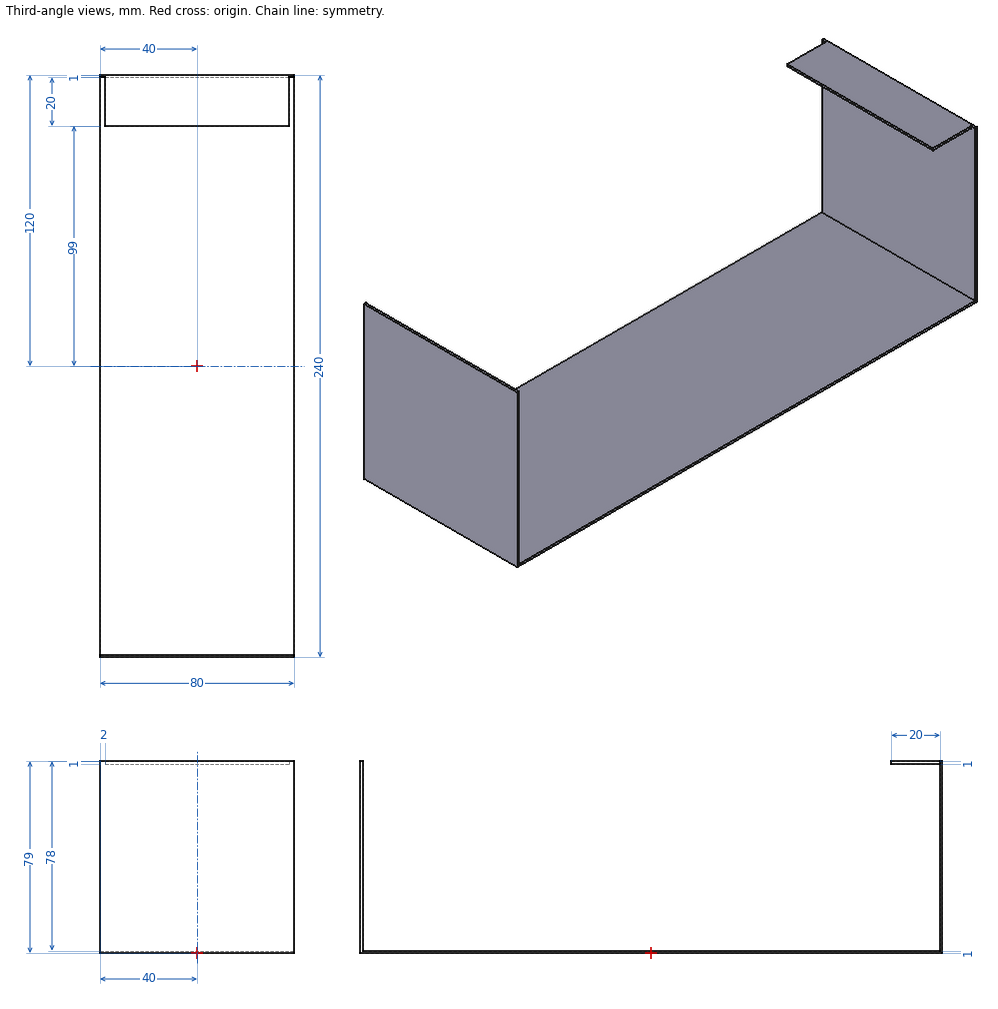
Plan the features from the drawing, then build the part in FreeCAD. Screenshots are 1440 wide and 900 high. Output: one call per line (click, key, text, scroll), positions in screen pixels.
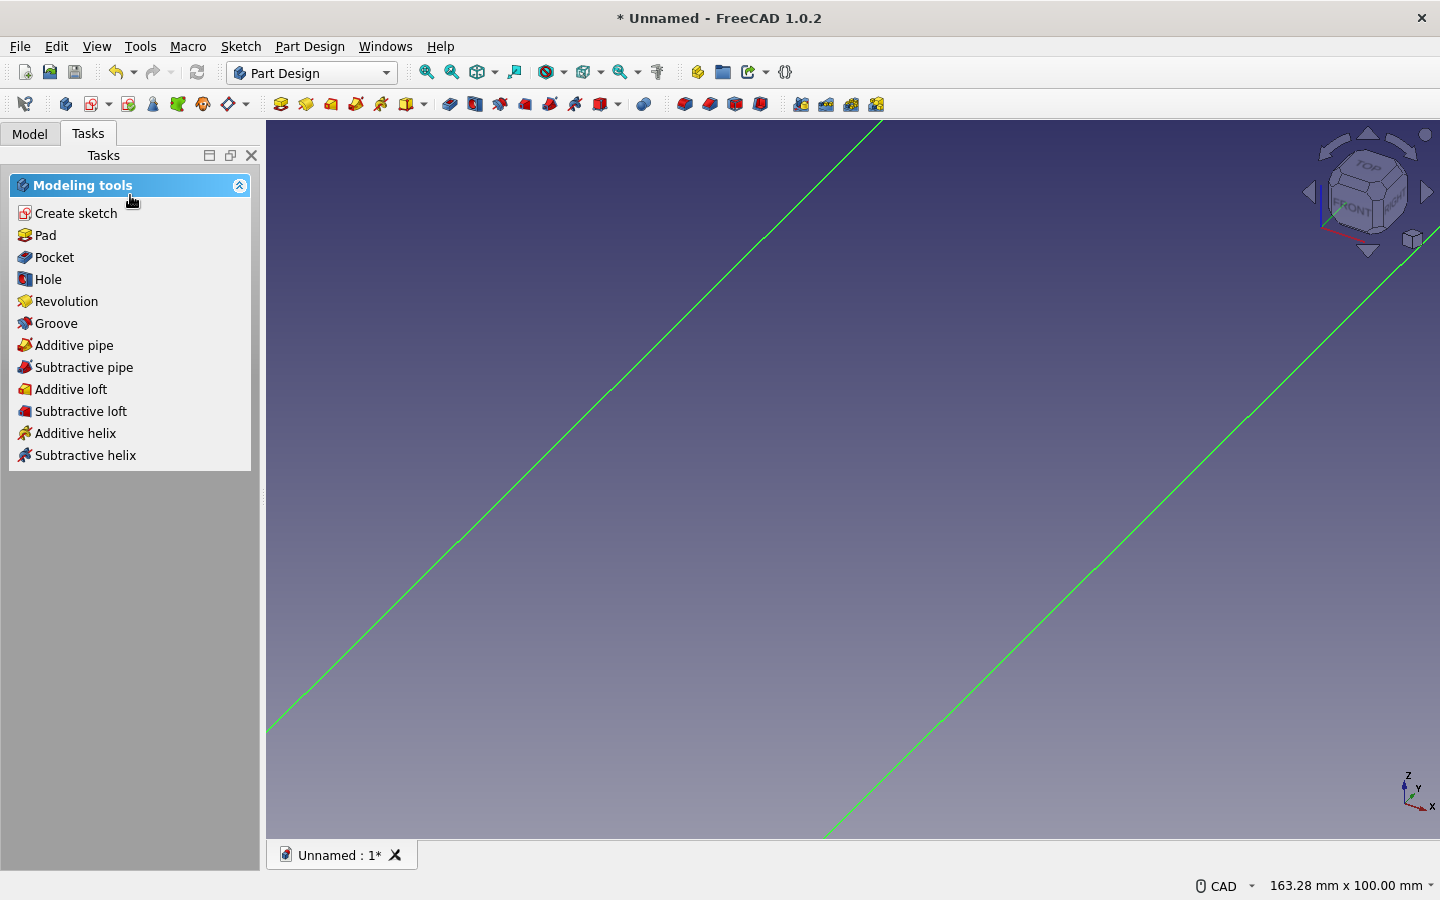
click(281, 104)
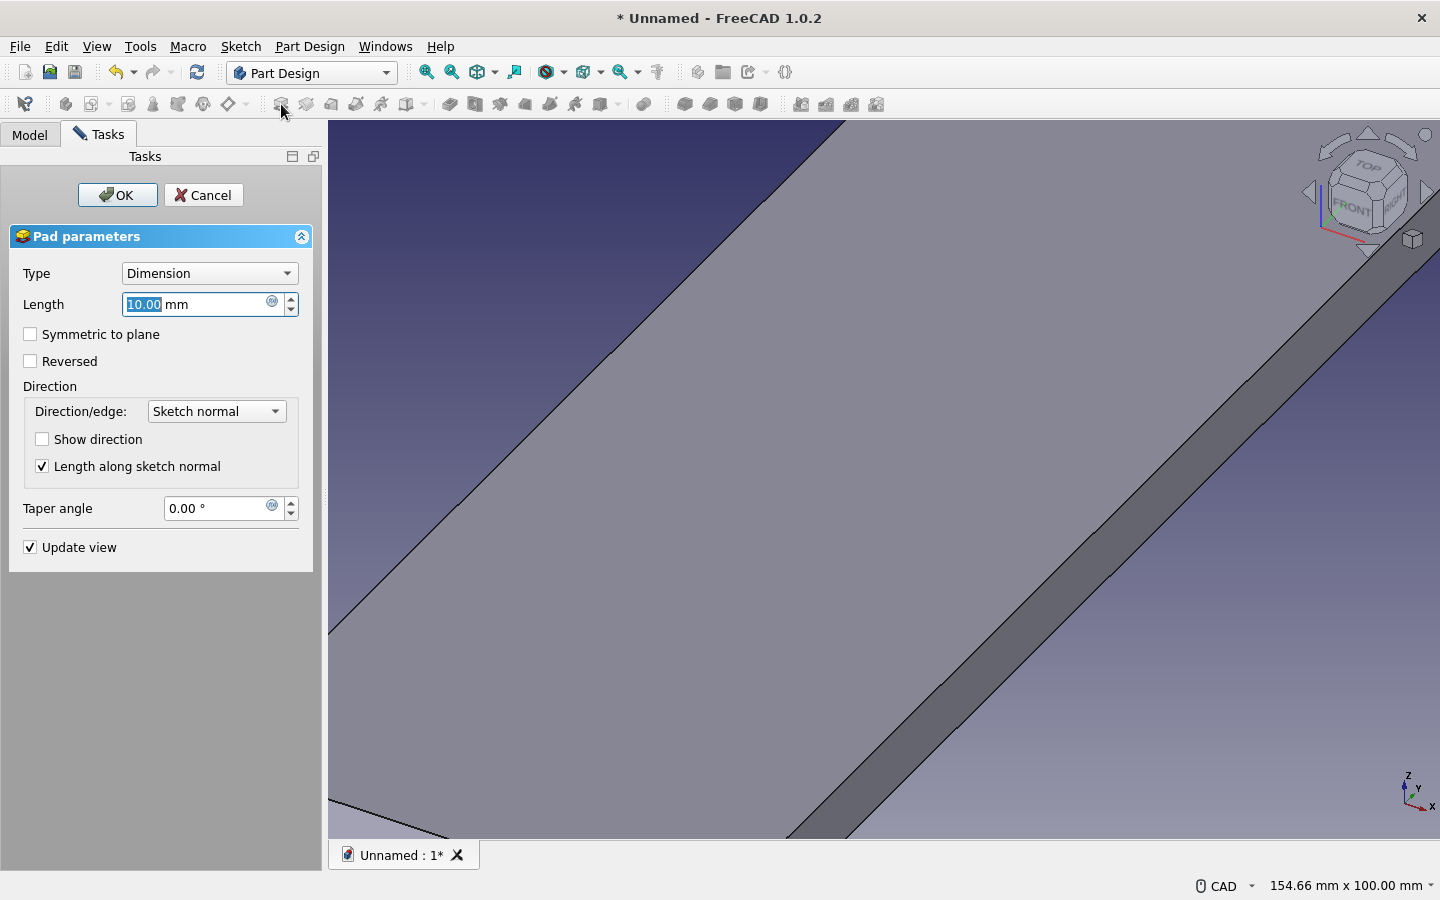
text(1)
key(Tab)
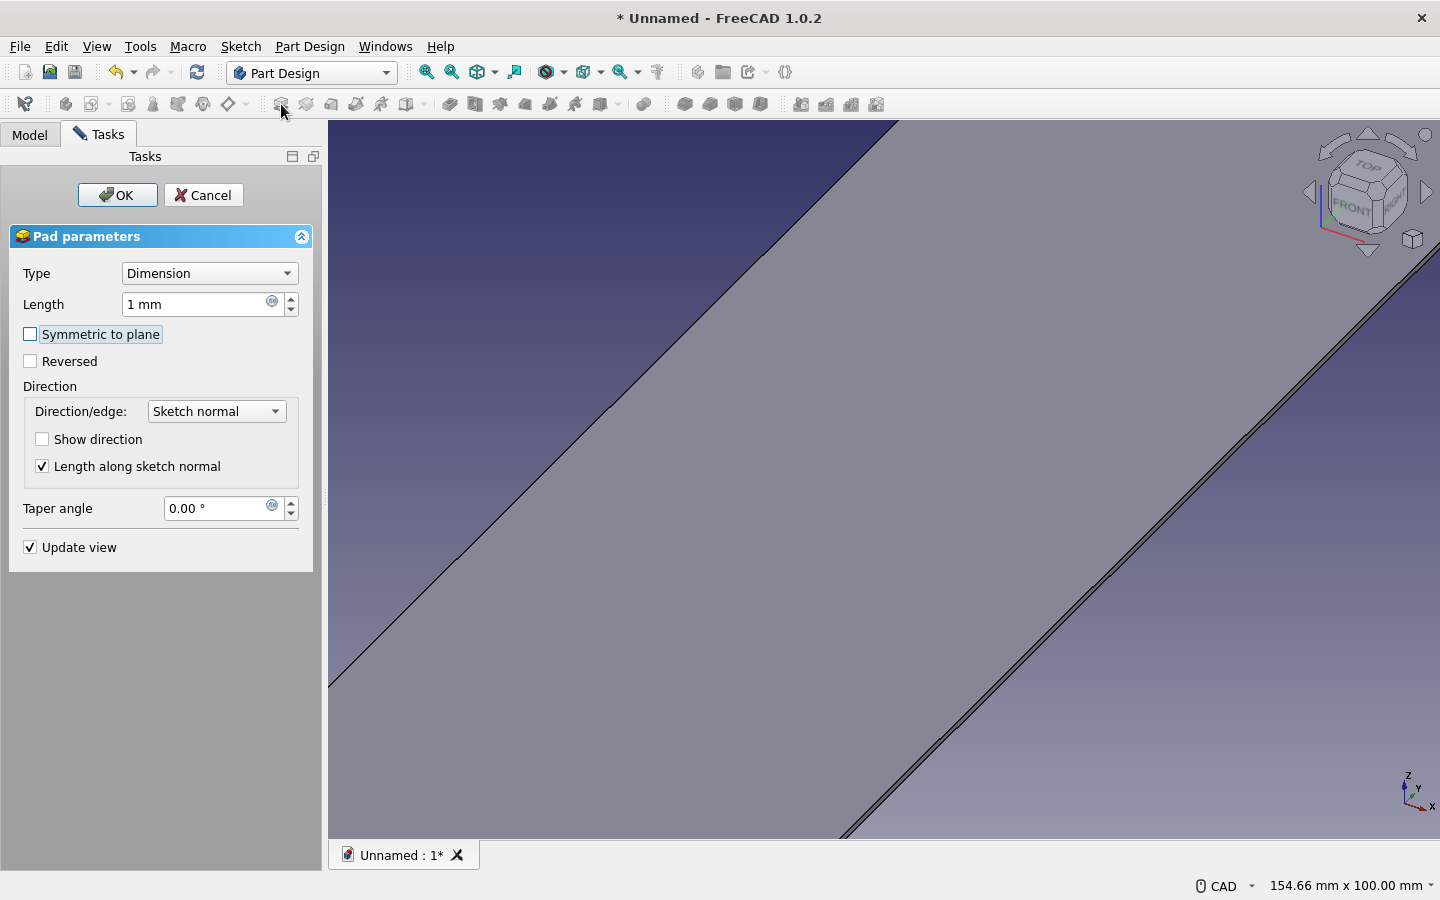
click(118, 195)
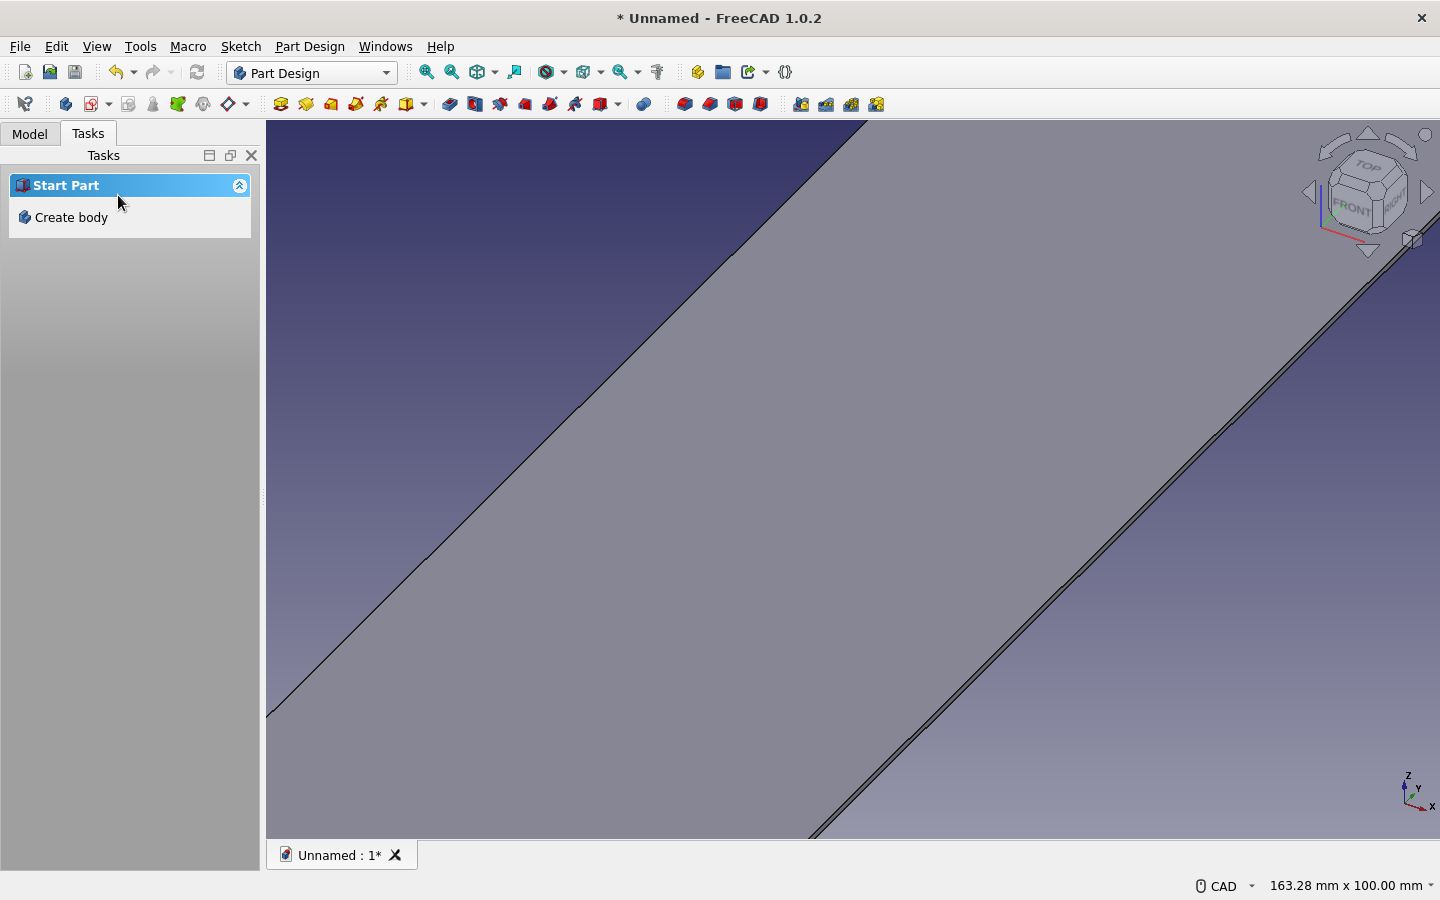
click(427, 72)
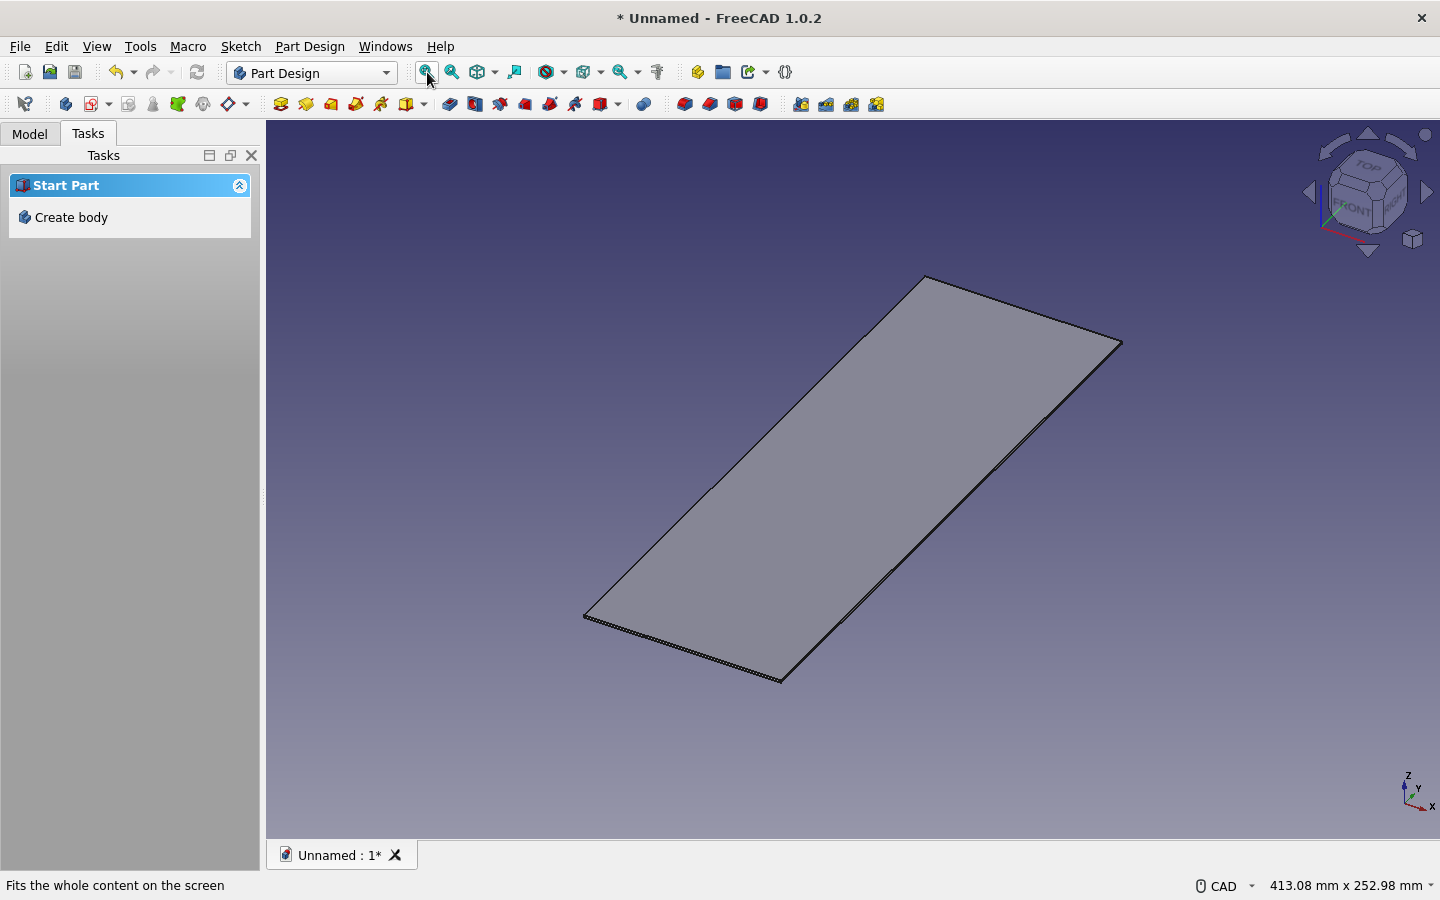
click(950, 381)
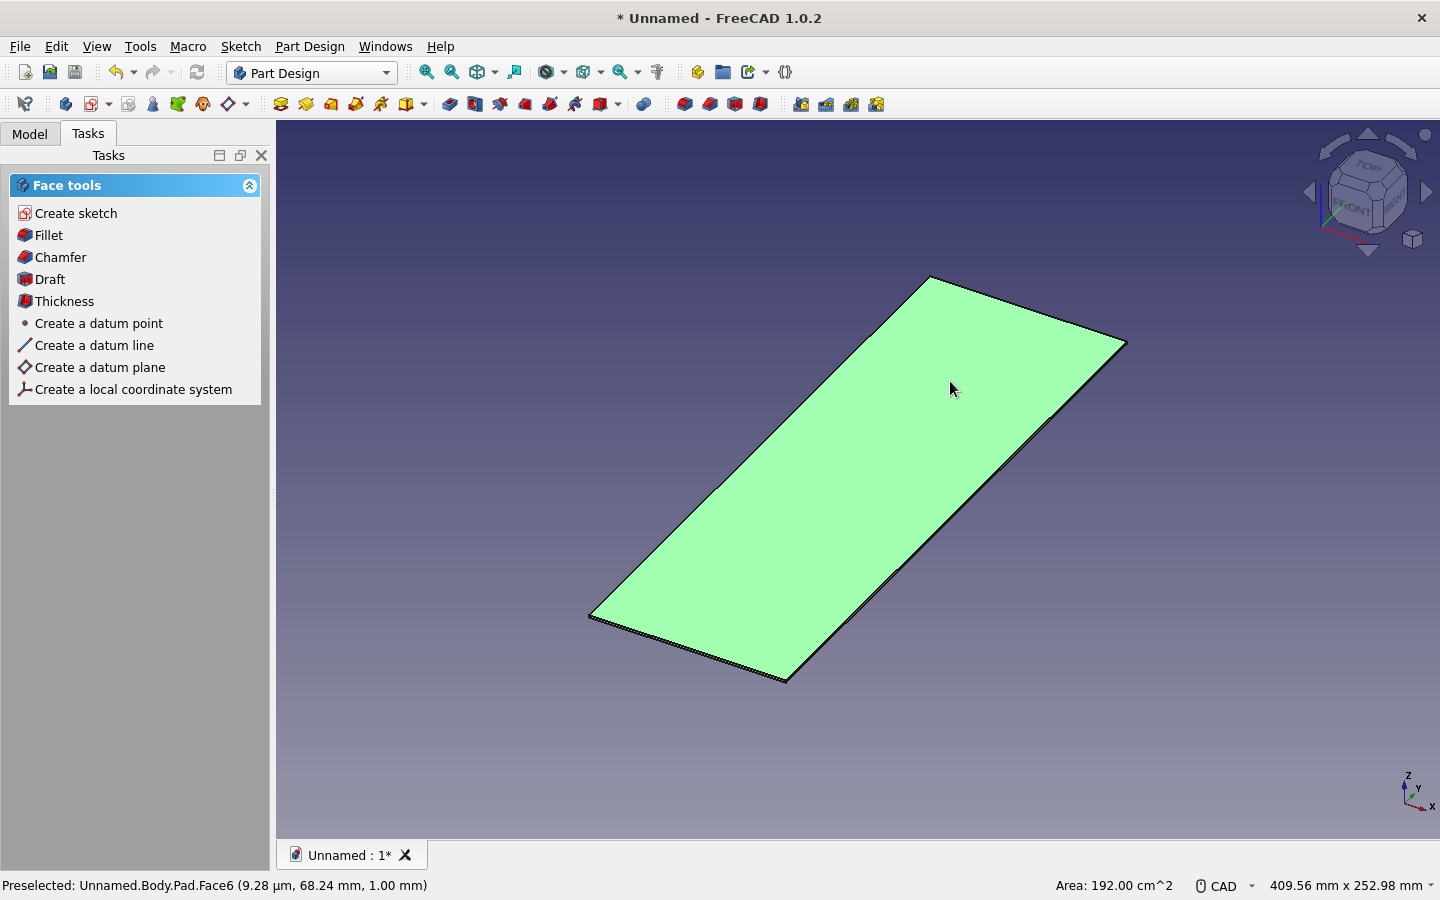
click(90, 104)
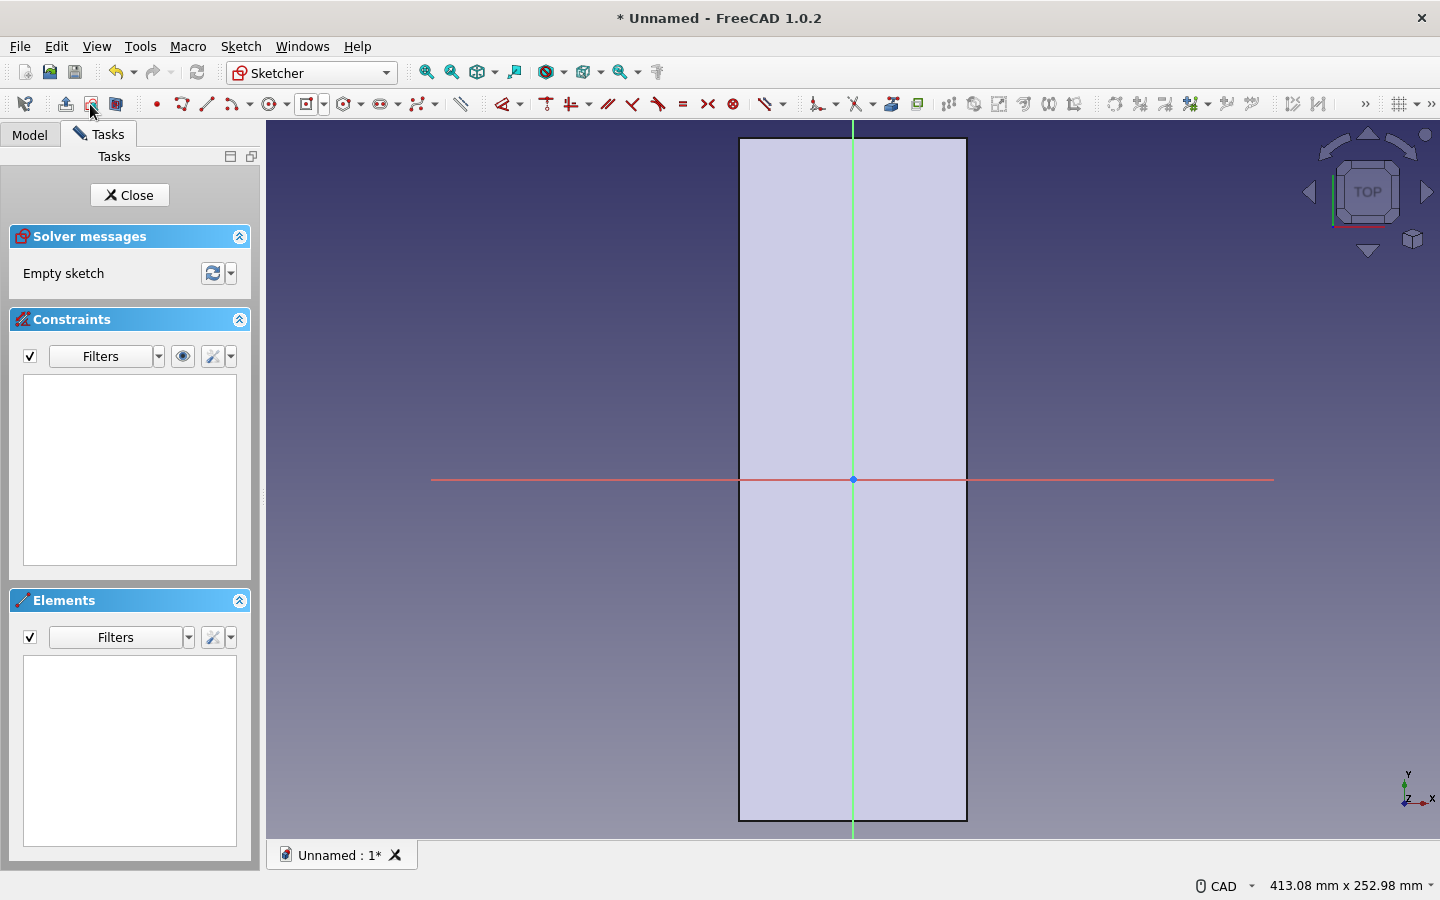
scroll(645, 480, down, 2)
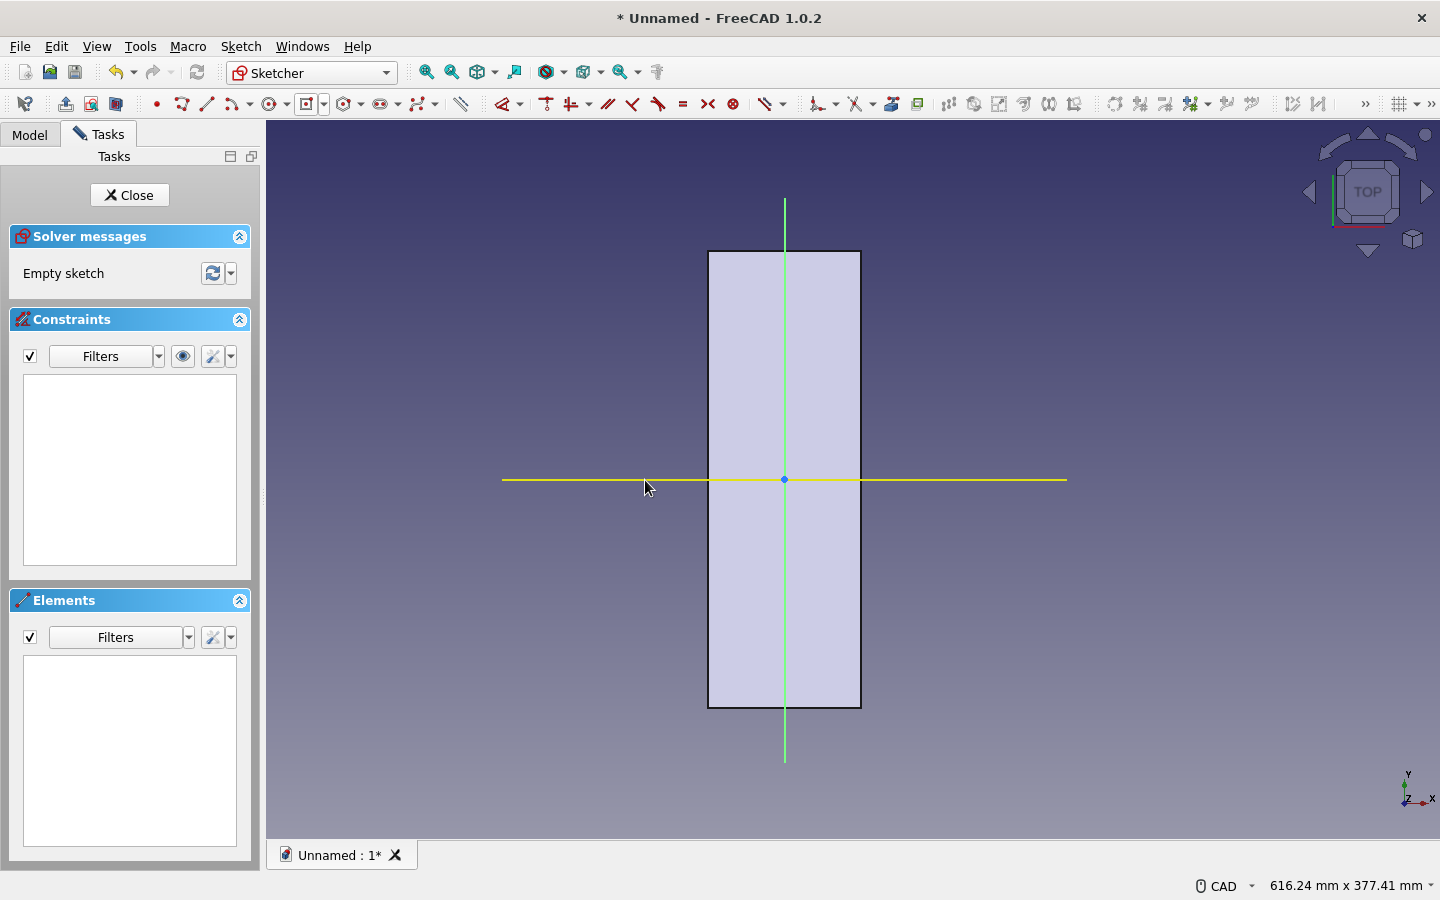
key(g)
key(r)